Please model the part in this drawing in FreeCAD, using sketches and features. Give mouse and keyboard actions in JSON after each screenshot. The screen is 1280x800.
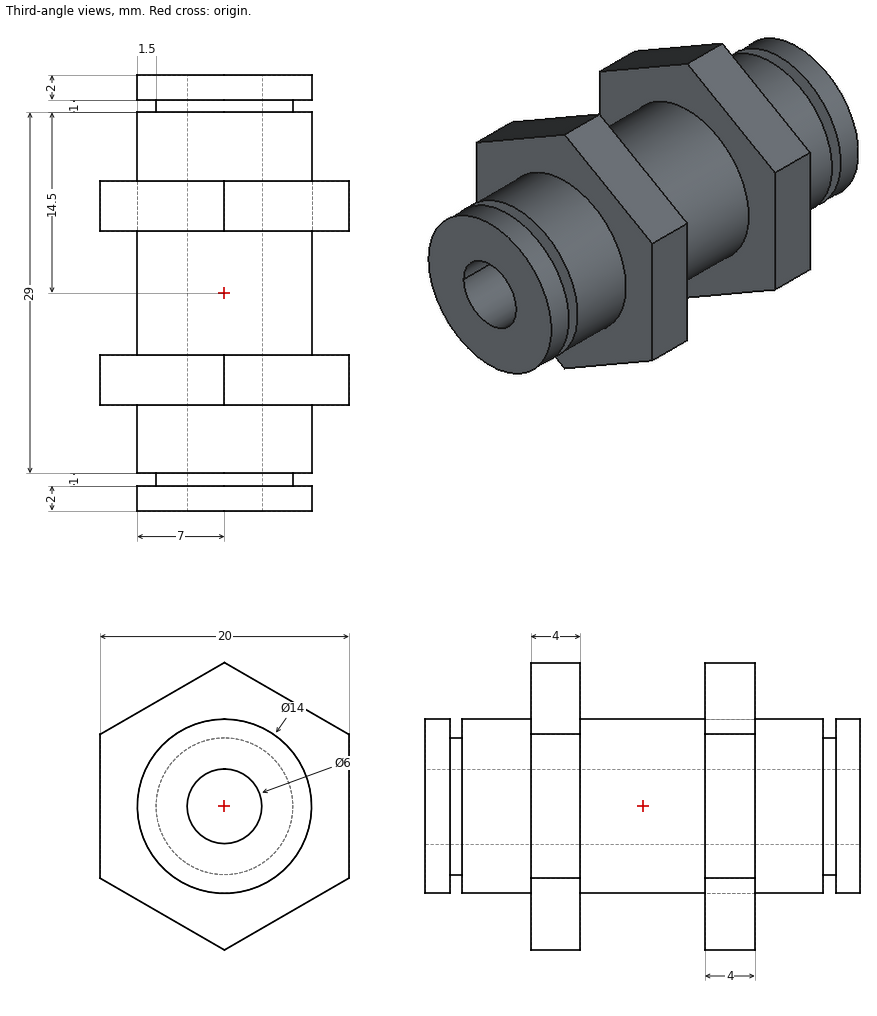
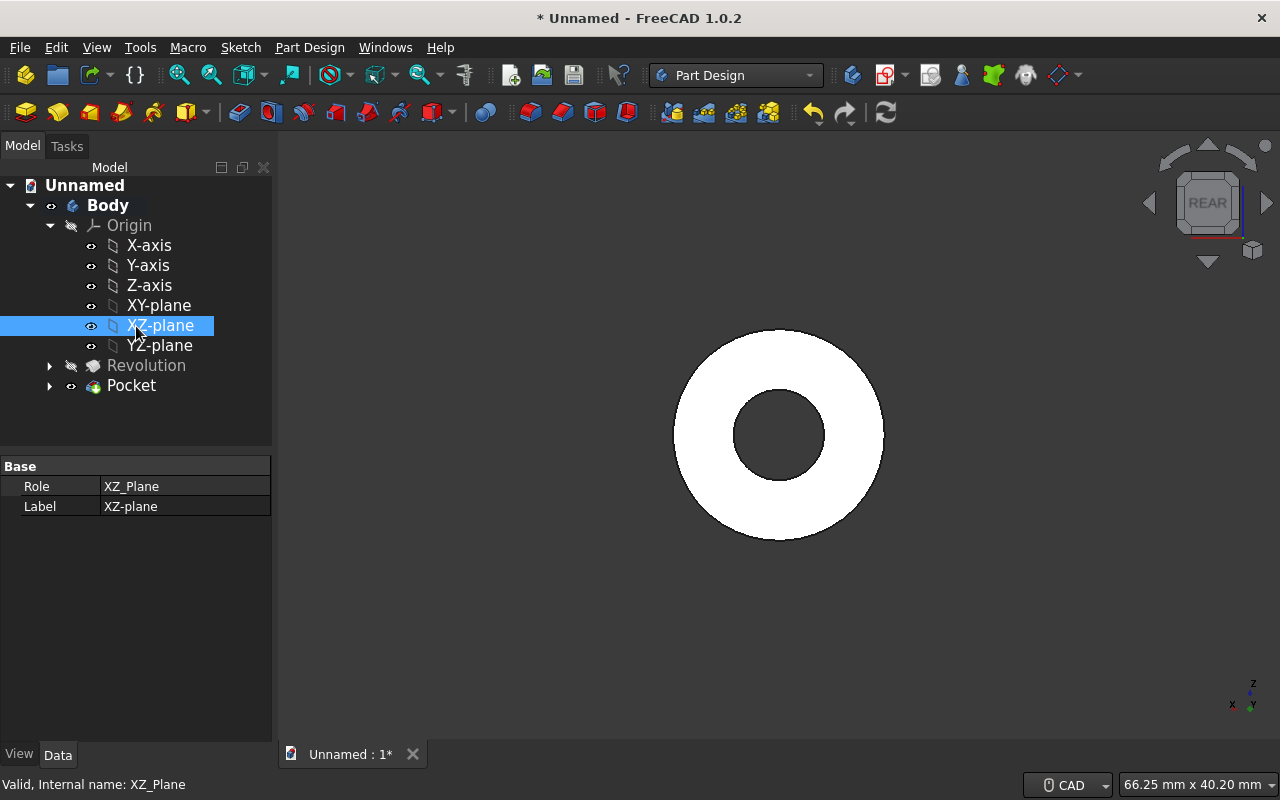
{"action": "left_click", "coordinate": [1058, 76]}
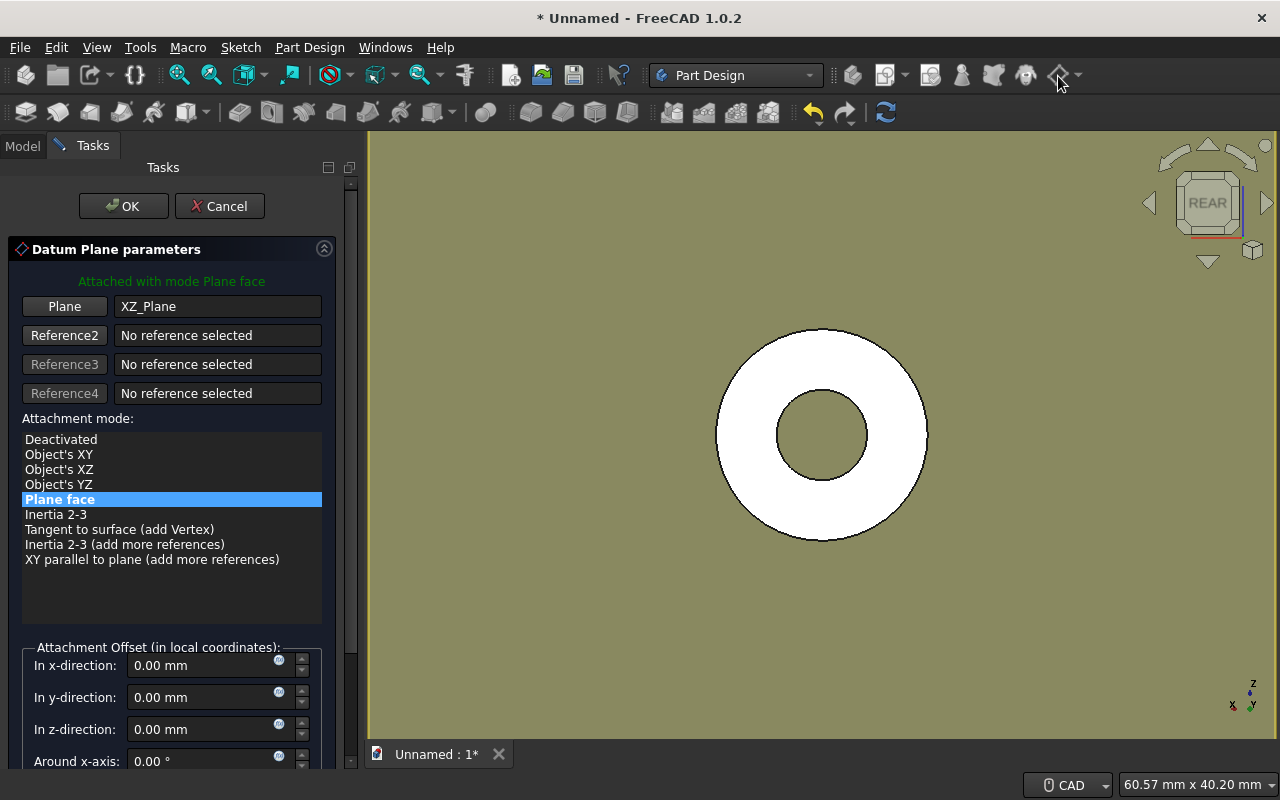
{"action": "triple_click", "coordinate": [210, 729]}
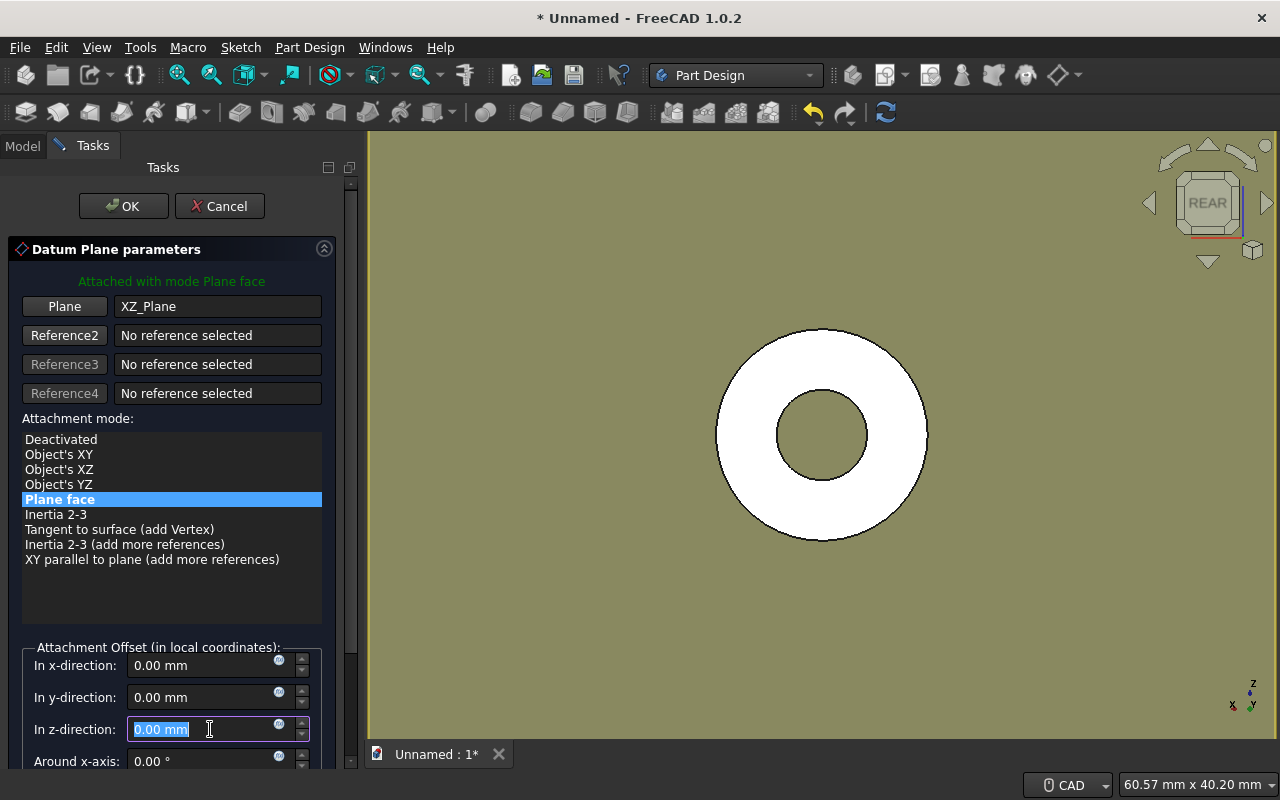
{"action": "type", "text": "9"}
{"action": "key", "text": "Tab"}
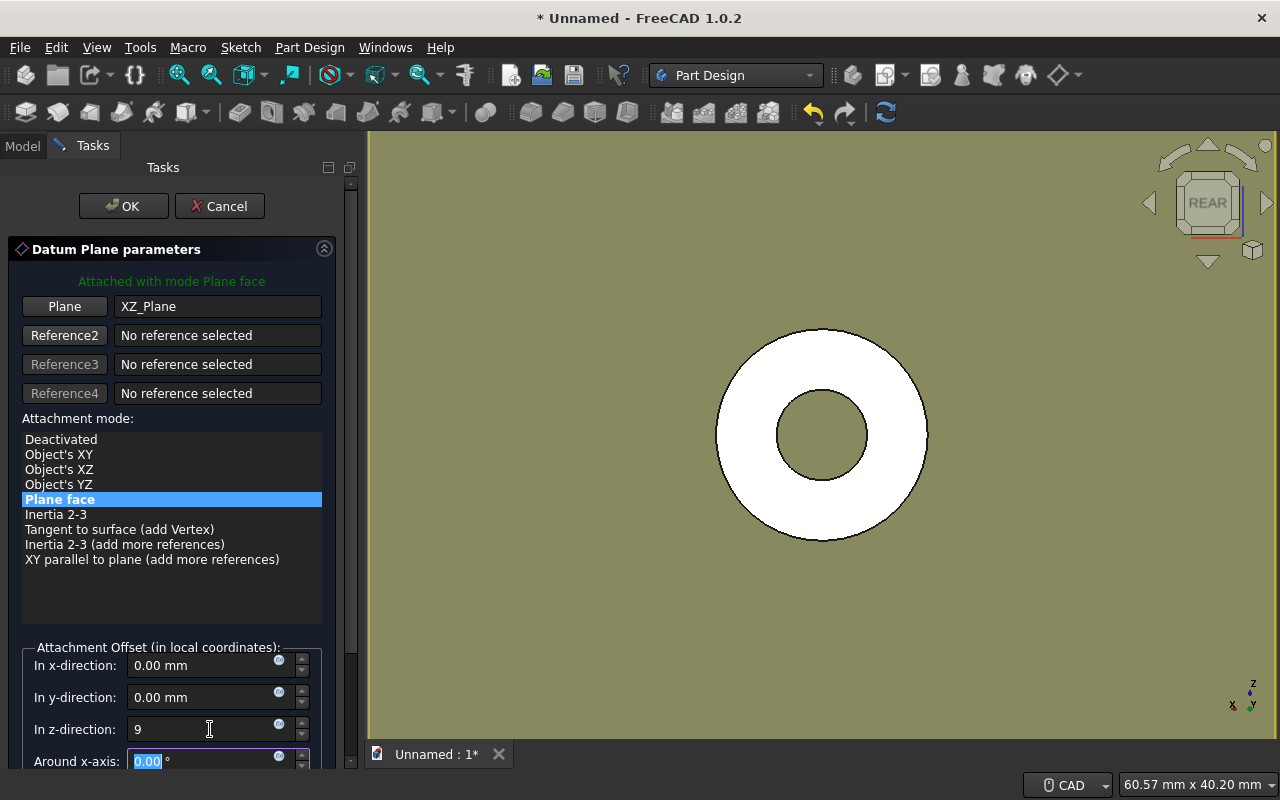
{"action": "left_click", "coordinate": [124, 206]}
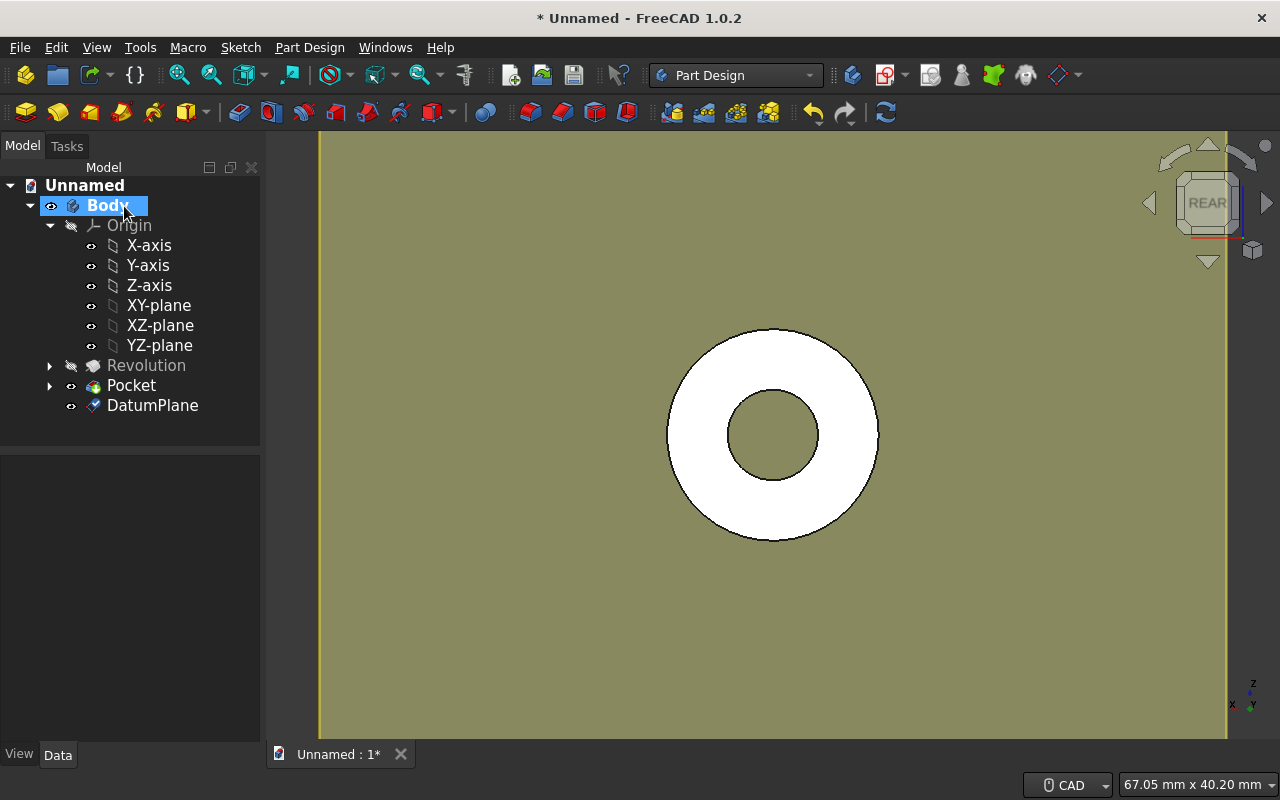
{"action": "left_click", "coordinate": [116, 406]}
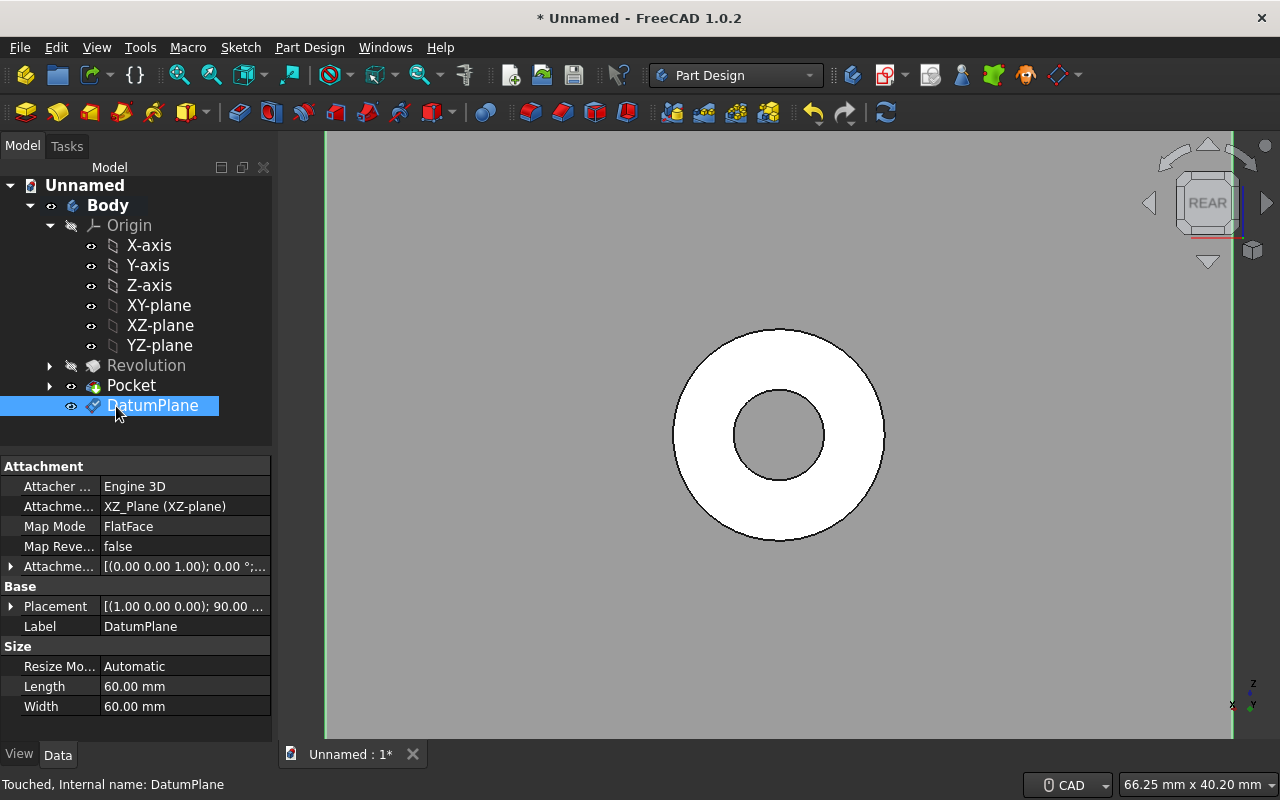
{"action": "left_click", "coordinate": [886, 76]}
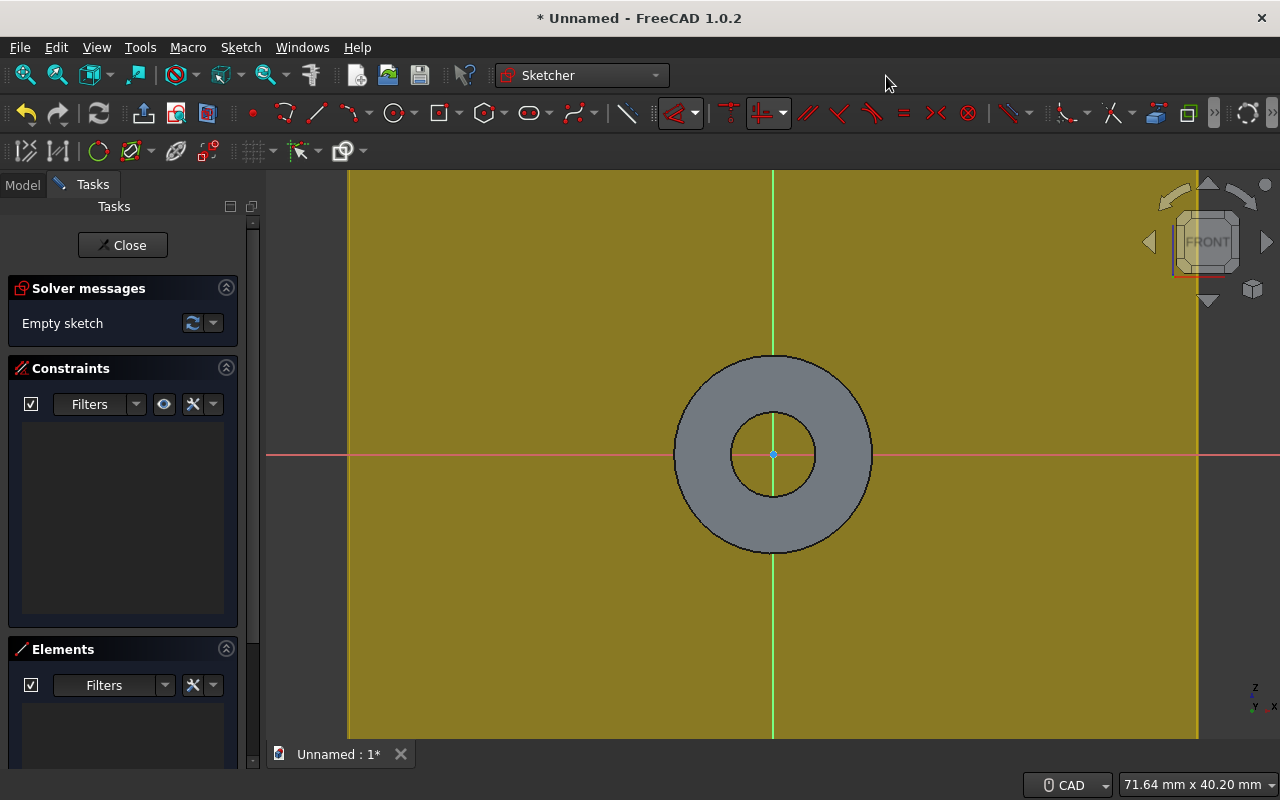
{"action": "left_click", "coordinate": [208, 114]}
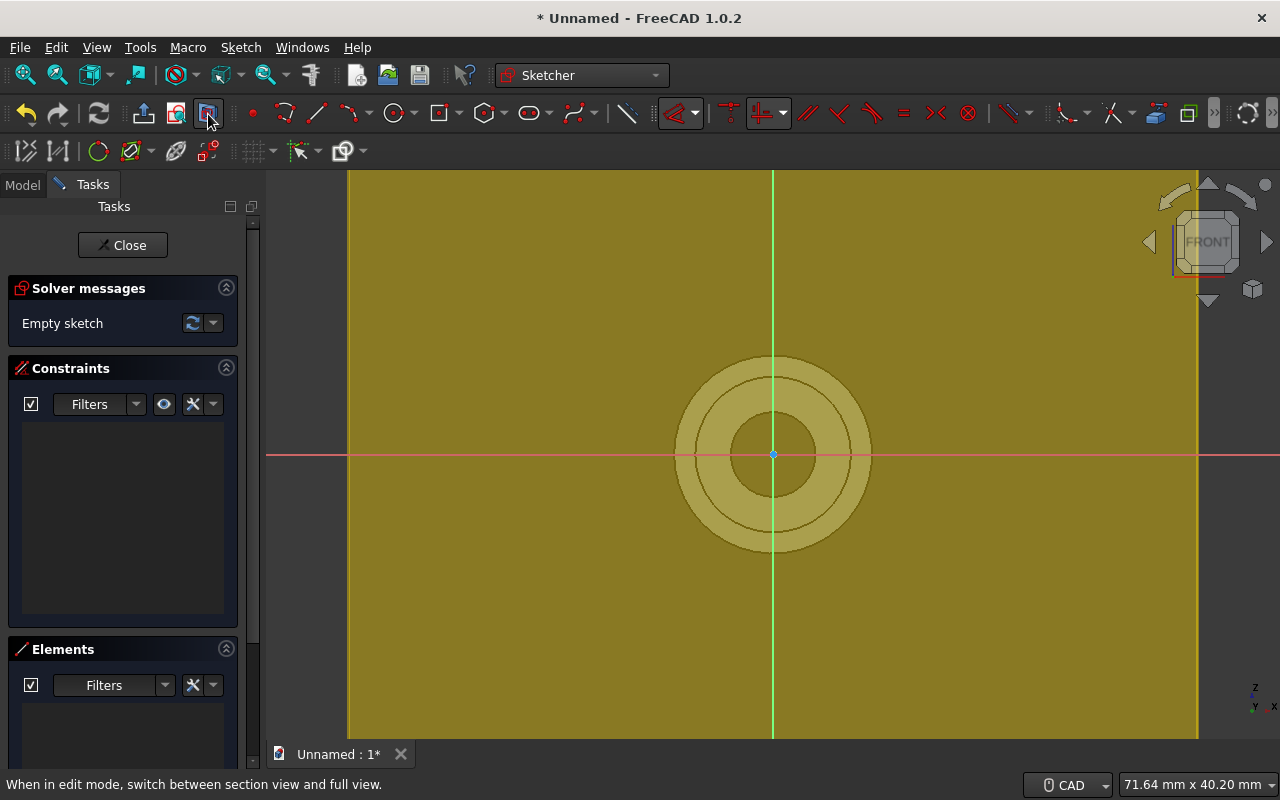
{"action": "left_click", "coordinate": [484, 114]}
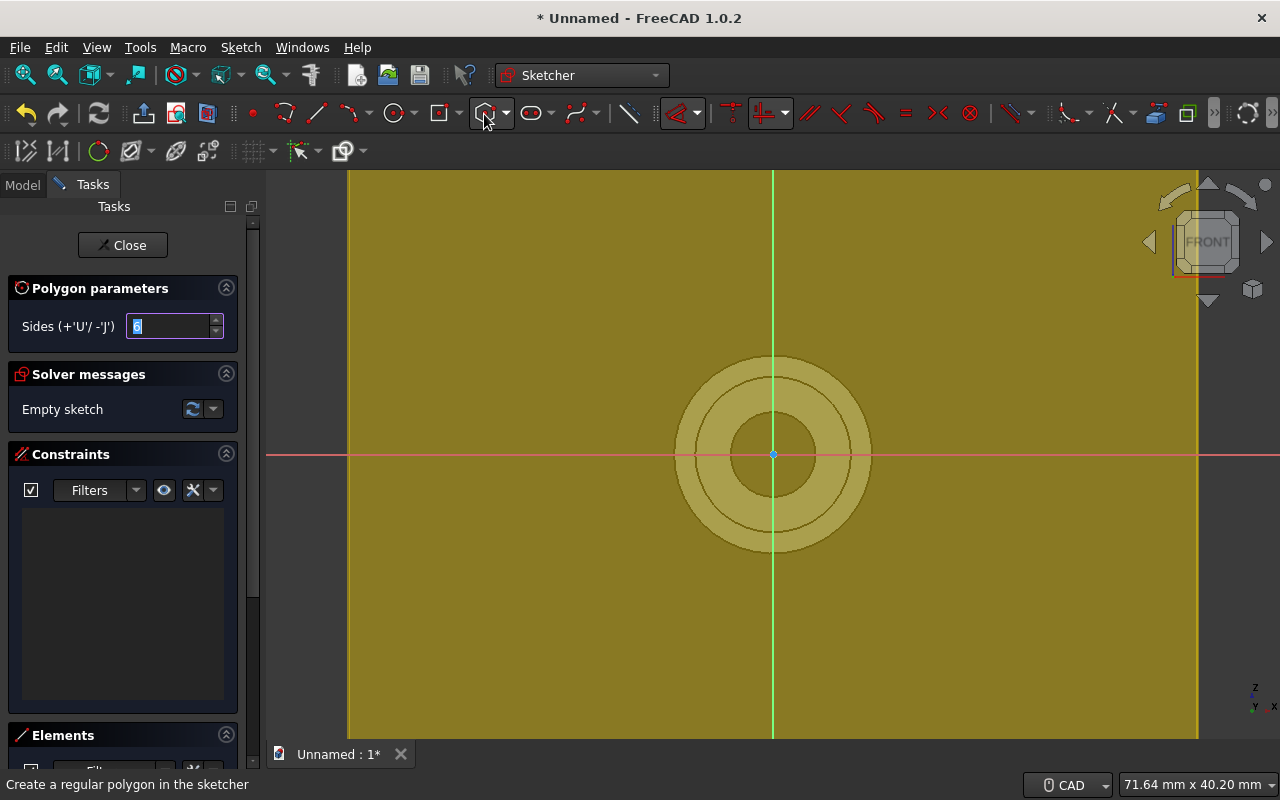
{"action": "left_click", "coordinate": [773, 455]}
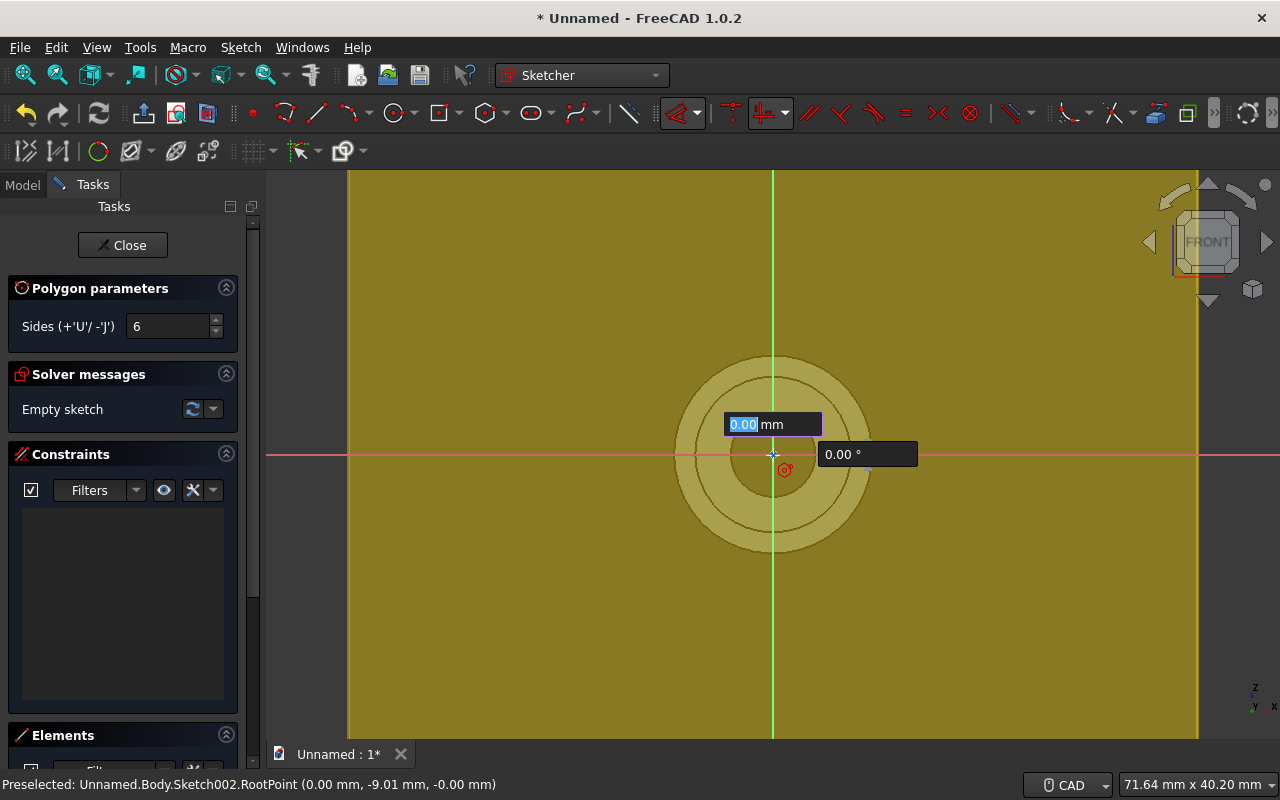
{"action": "left_click", "coordinate": [773, 618]}
{"action": "key", "text": "Escape"}